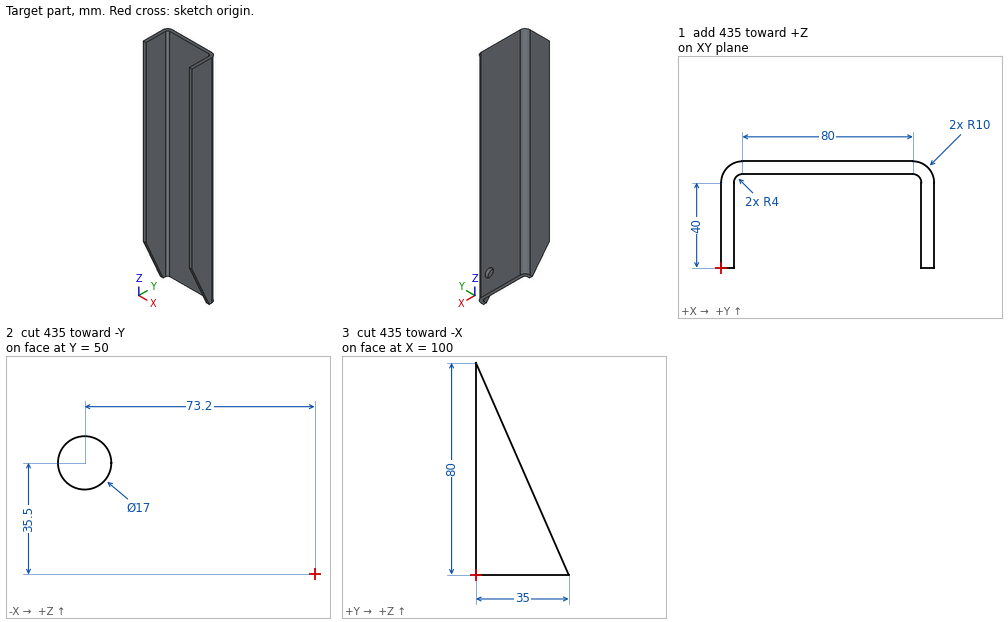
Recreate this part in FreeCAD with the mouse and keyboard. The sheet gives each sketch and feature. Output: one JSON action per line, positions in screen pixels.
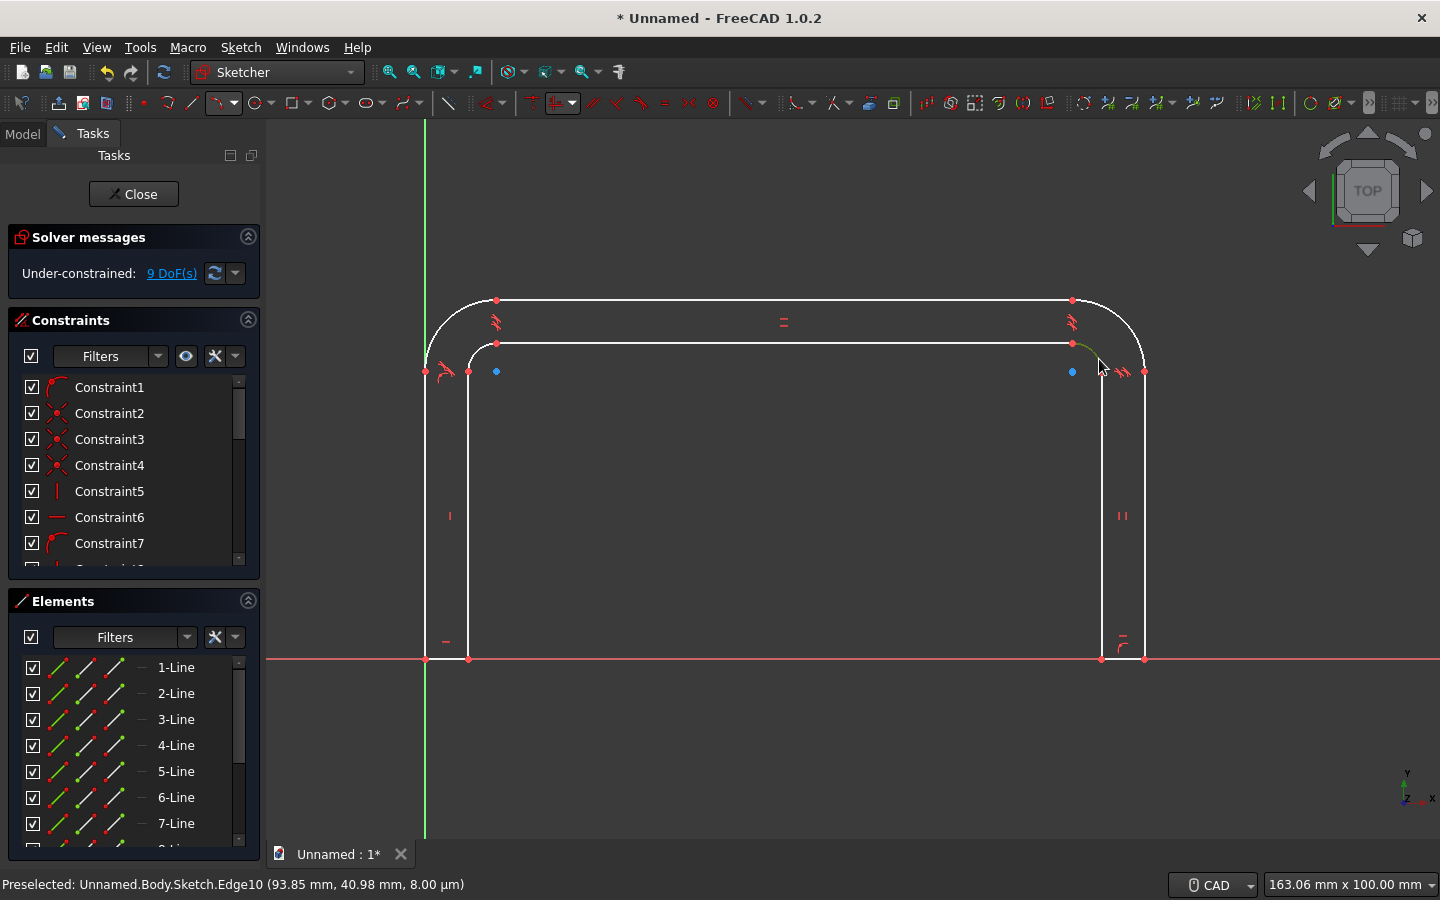
{"action": "left_click", "coordinate": [1137, 339]}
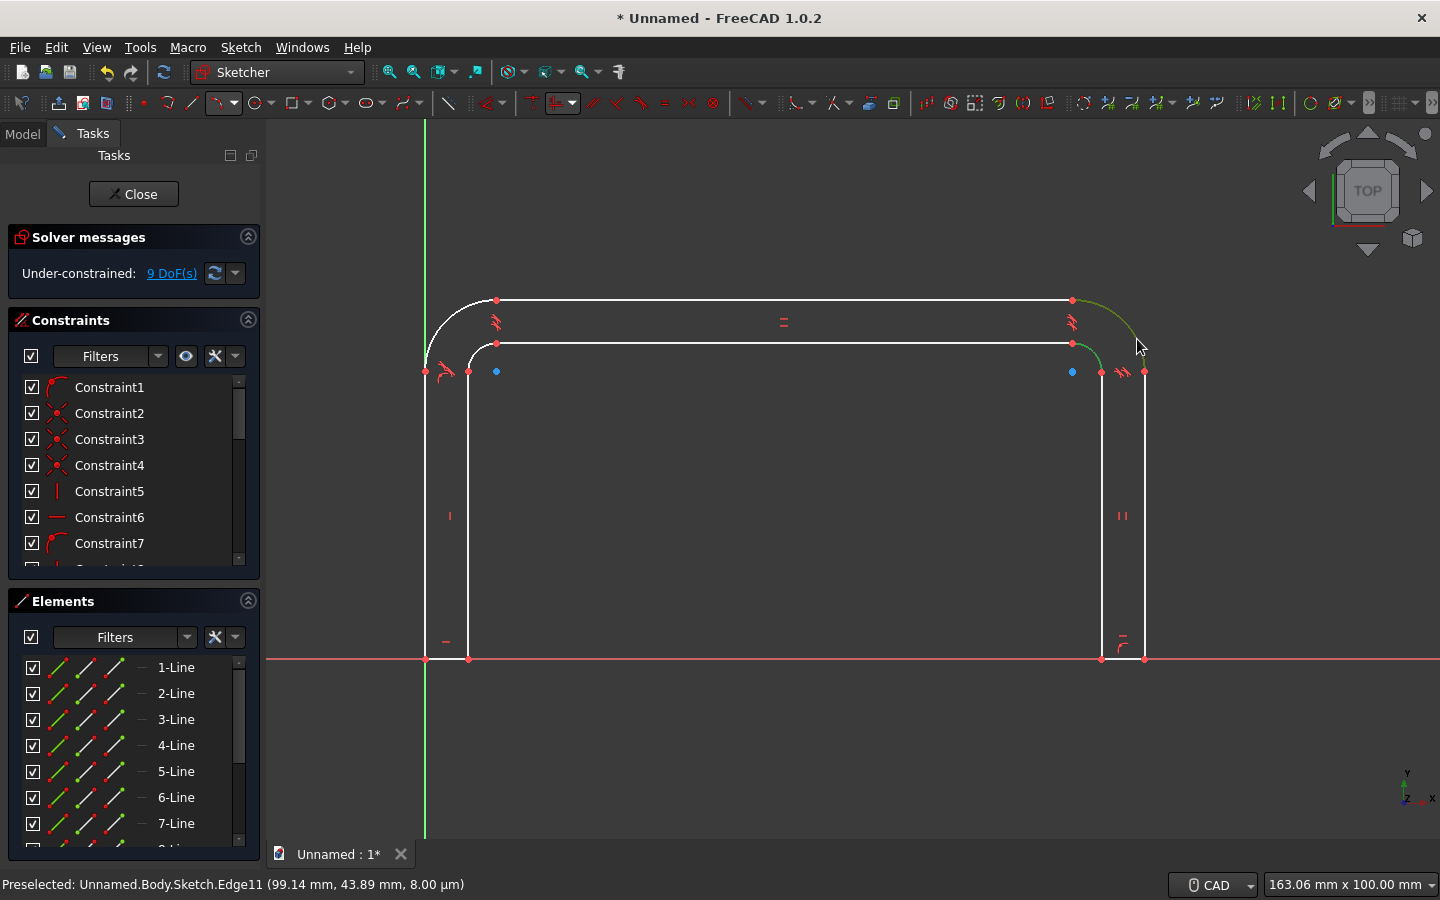
{"action": "left_click", "coordinate": [532, 104]}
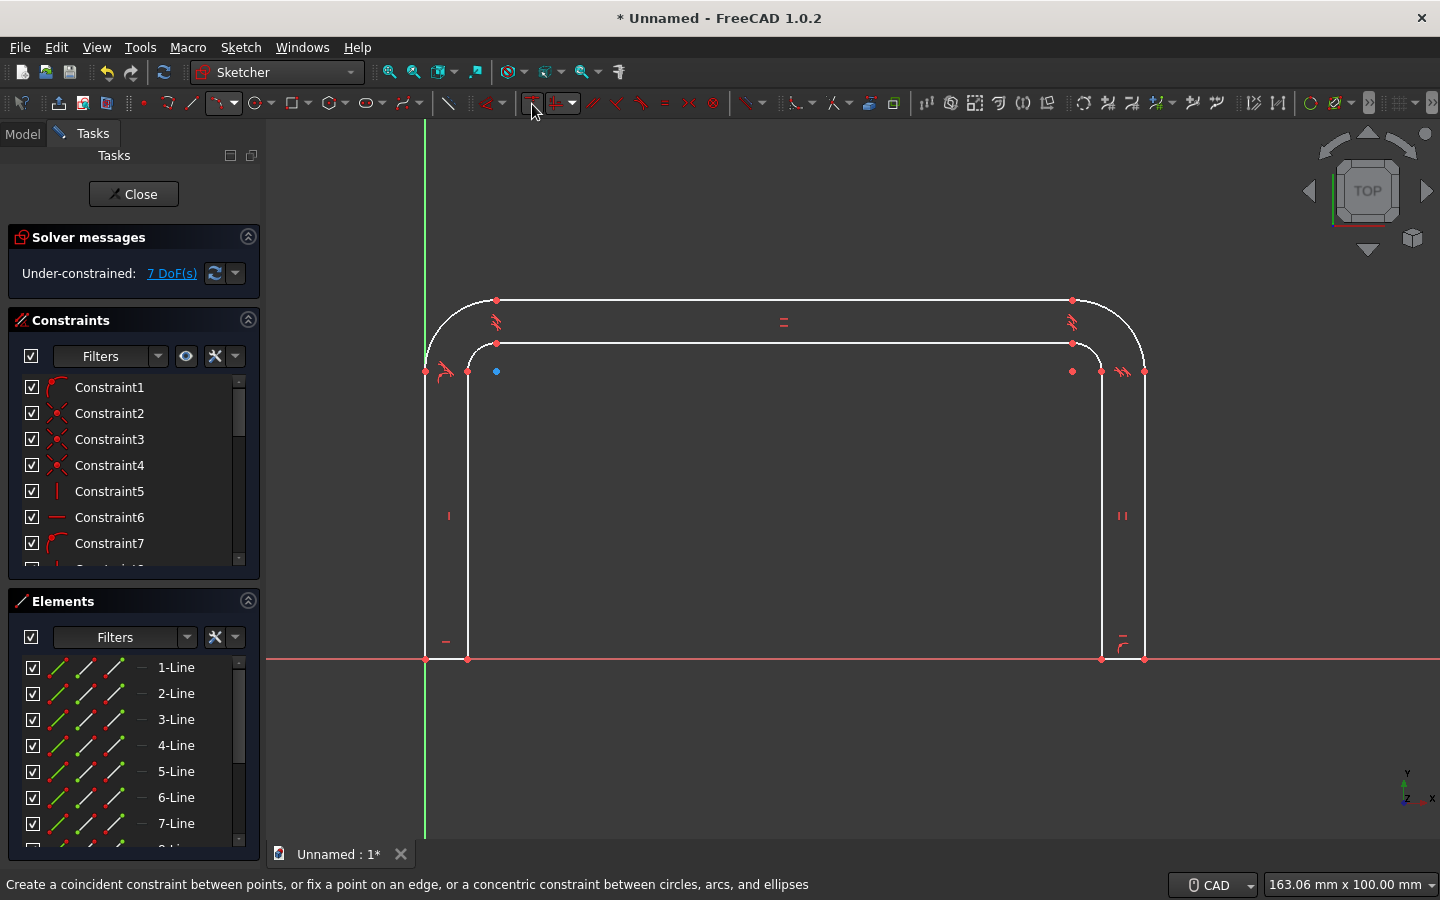
{"action": "left_click", "coordinate": [484, 346]}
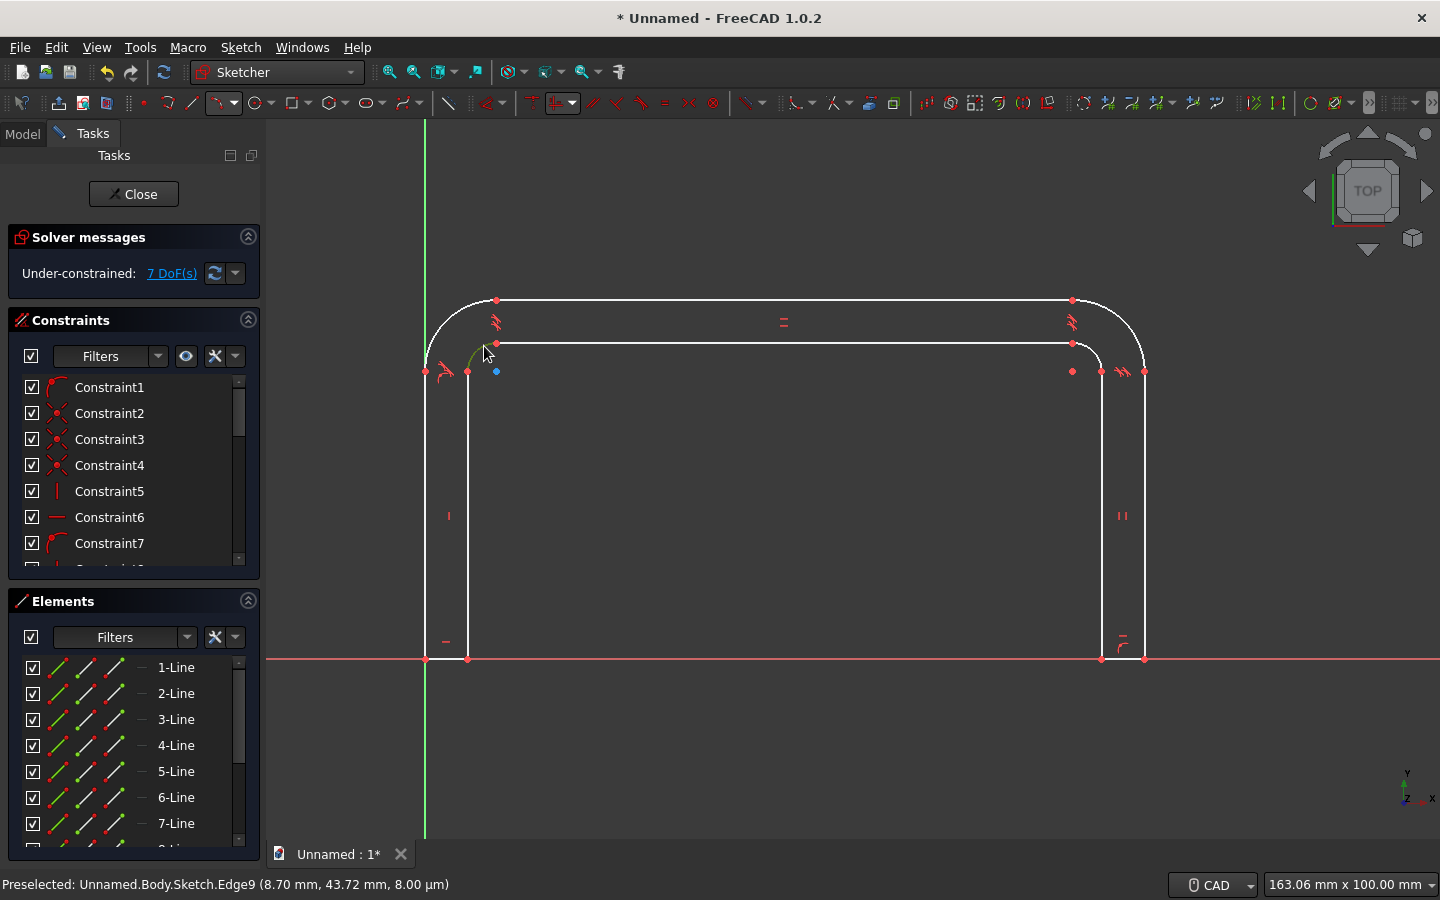
{"action": "left_click", "coordinate": [464, 308]}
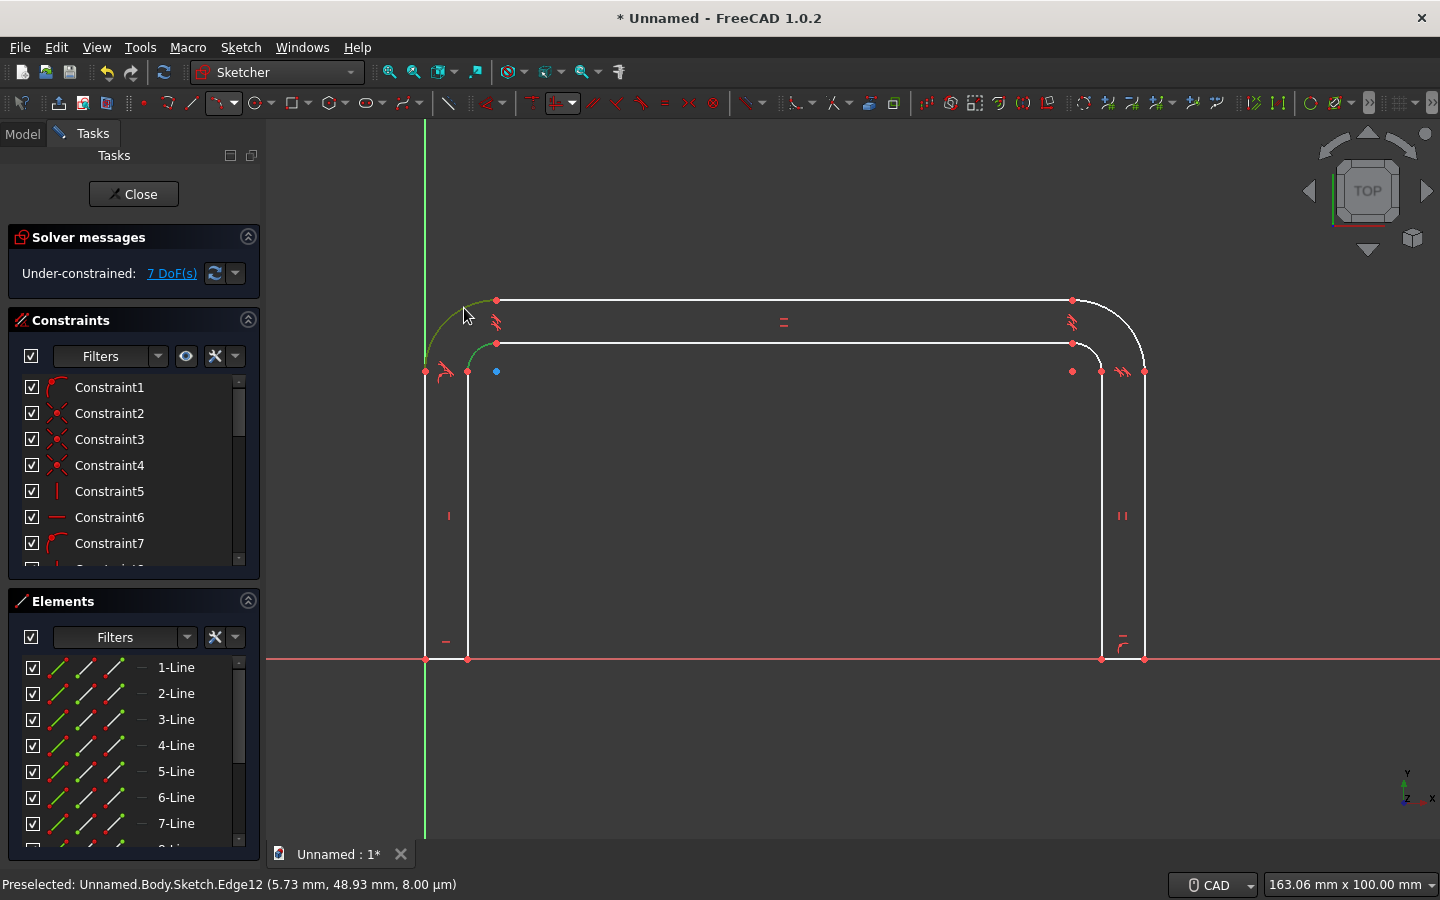
{"action": "left_click", "coordinate": [532, 104]}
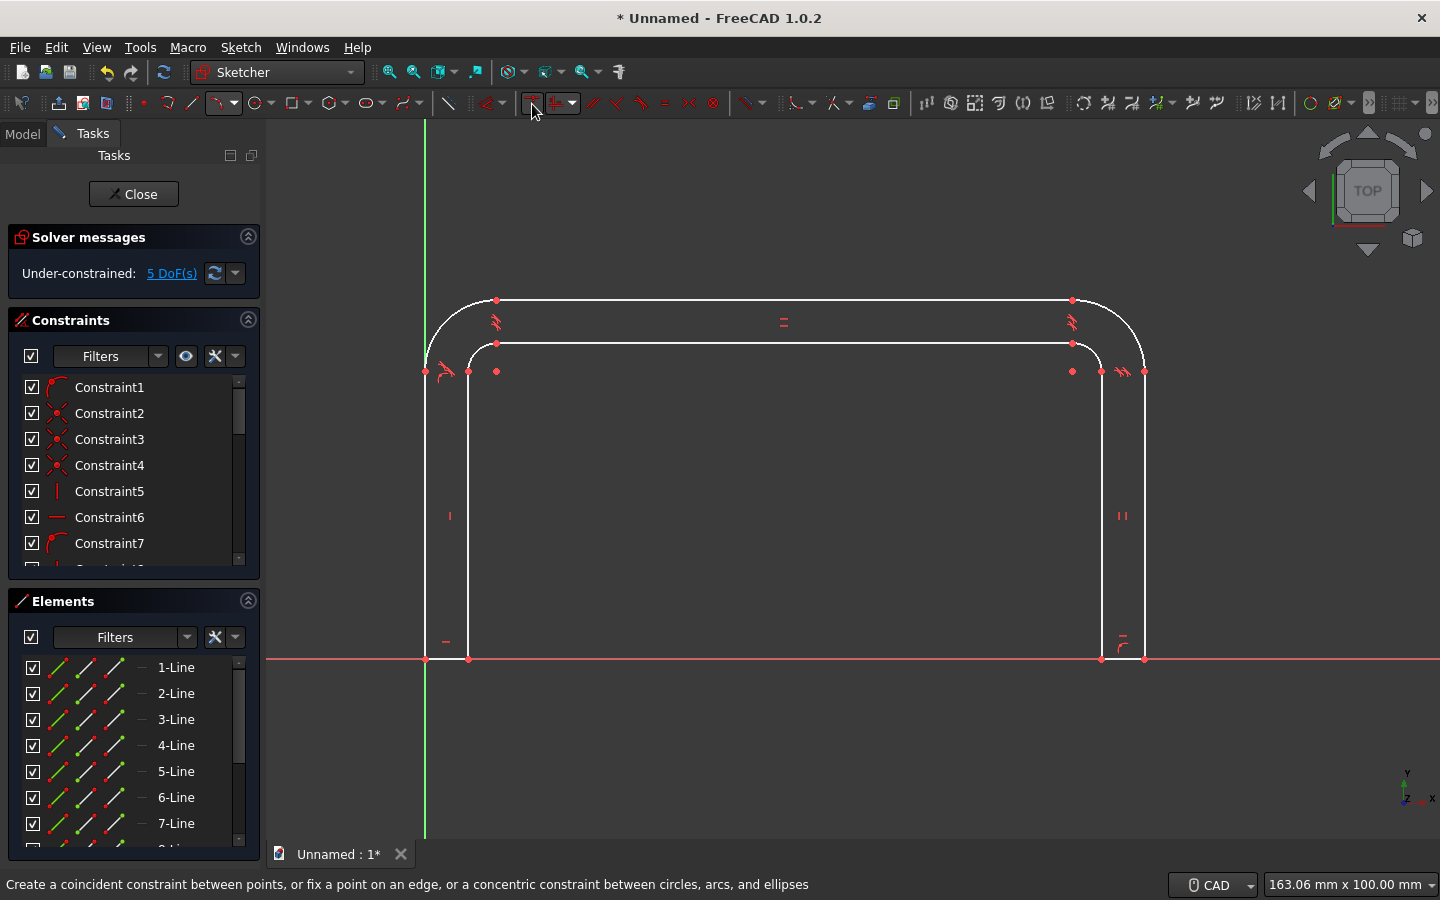
{"action": "left_click", "coordinate": [484, 346]}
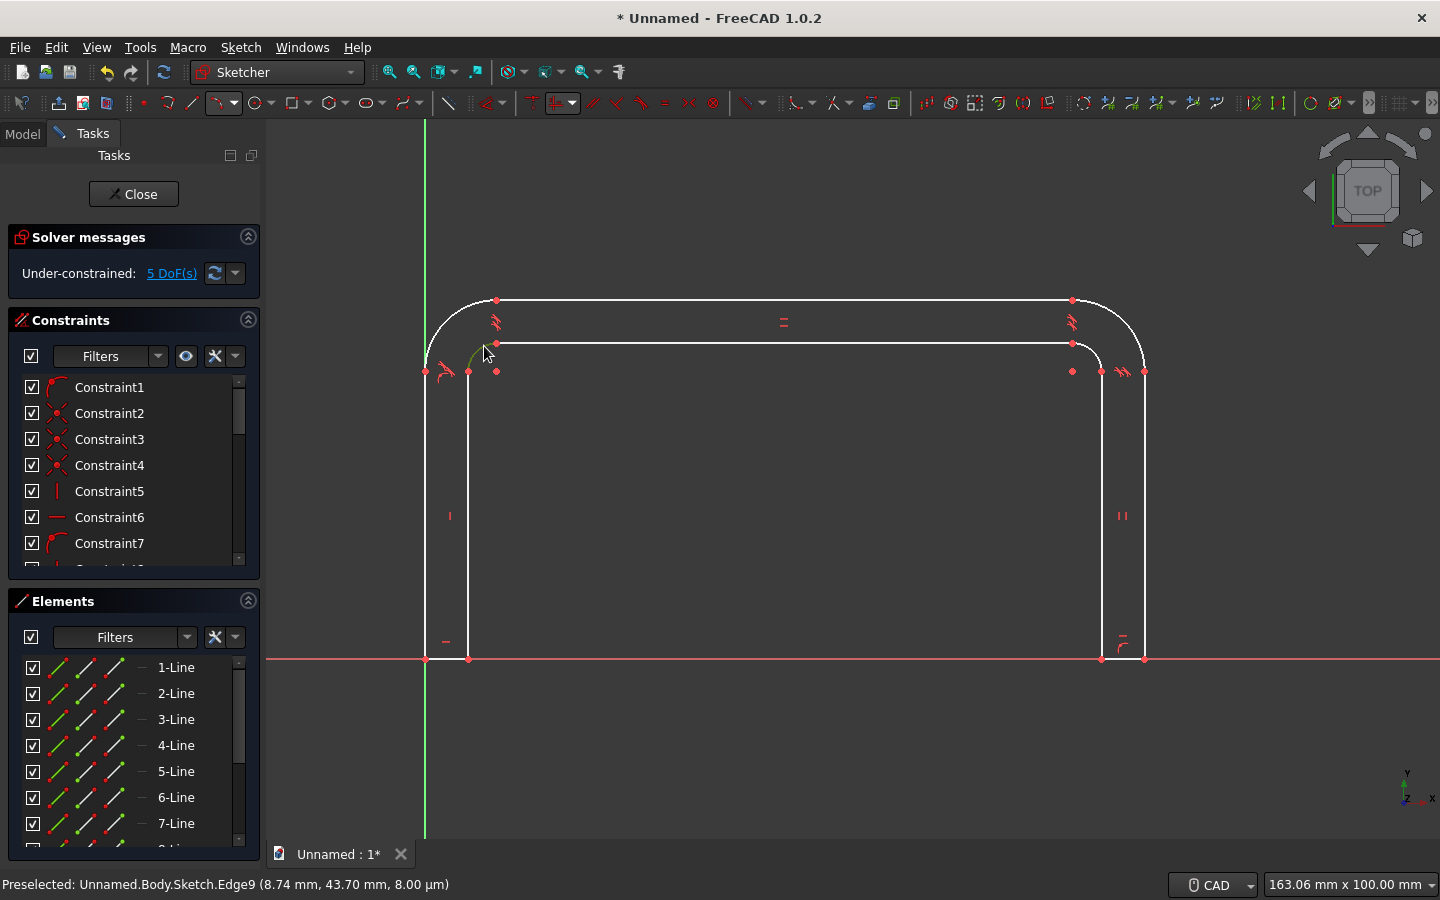
{"action": "left_click", "coordinate": [1099, 359]}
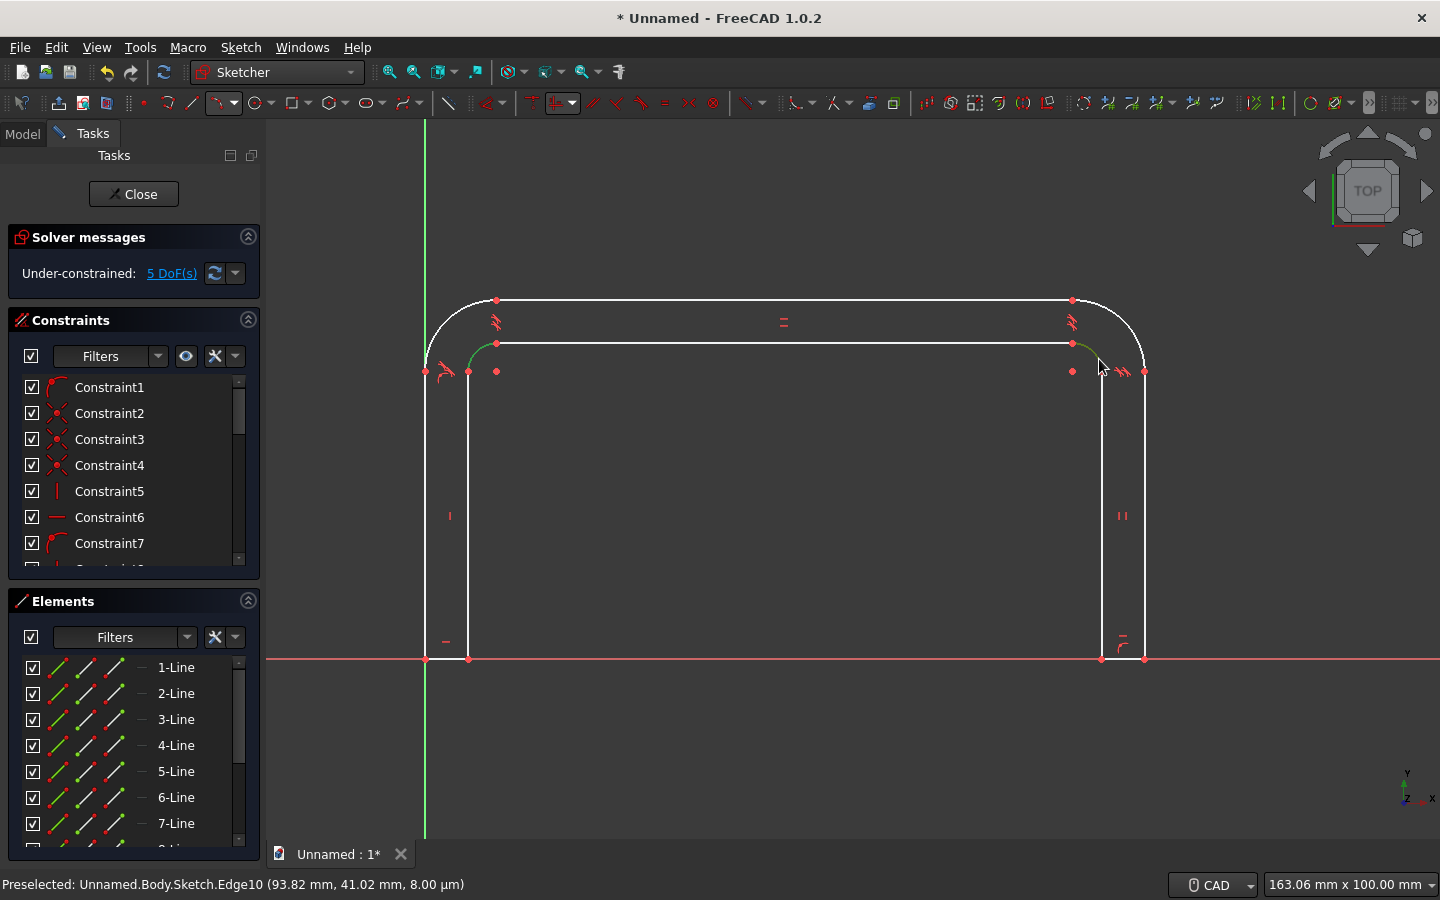
{"action": "left_click", "coordinate": [666, 104]}